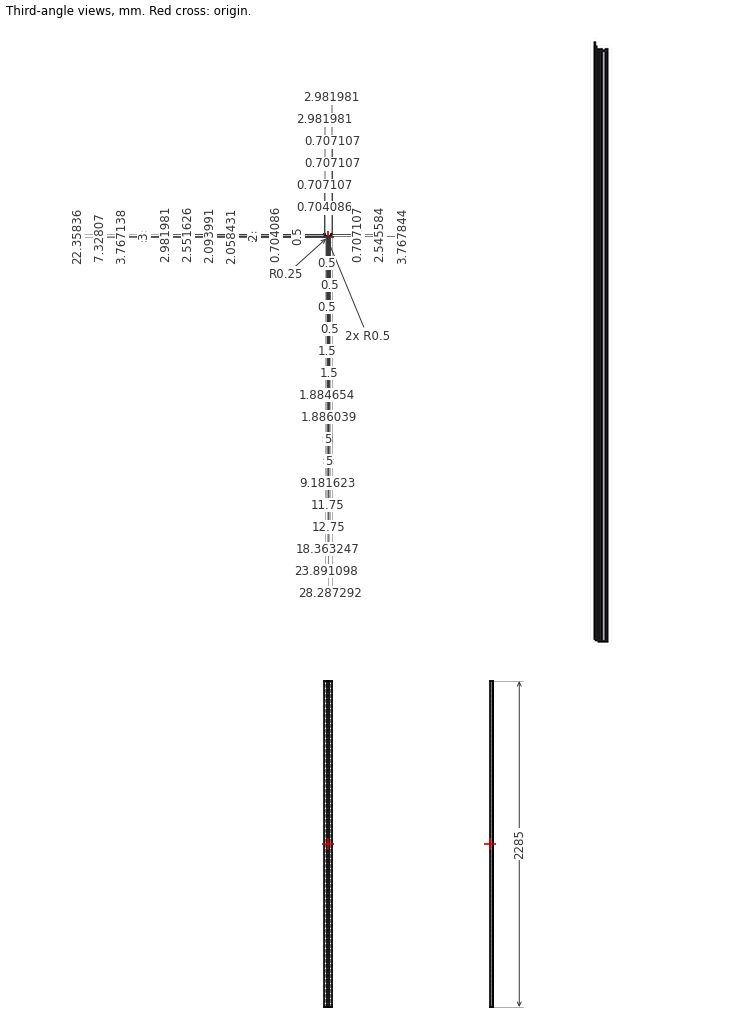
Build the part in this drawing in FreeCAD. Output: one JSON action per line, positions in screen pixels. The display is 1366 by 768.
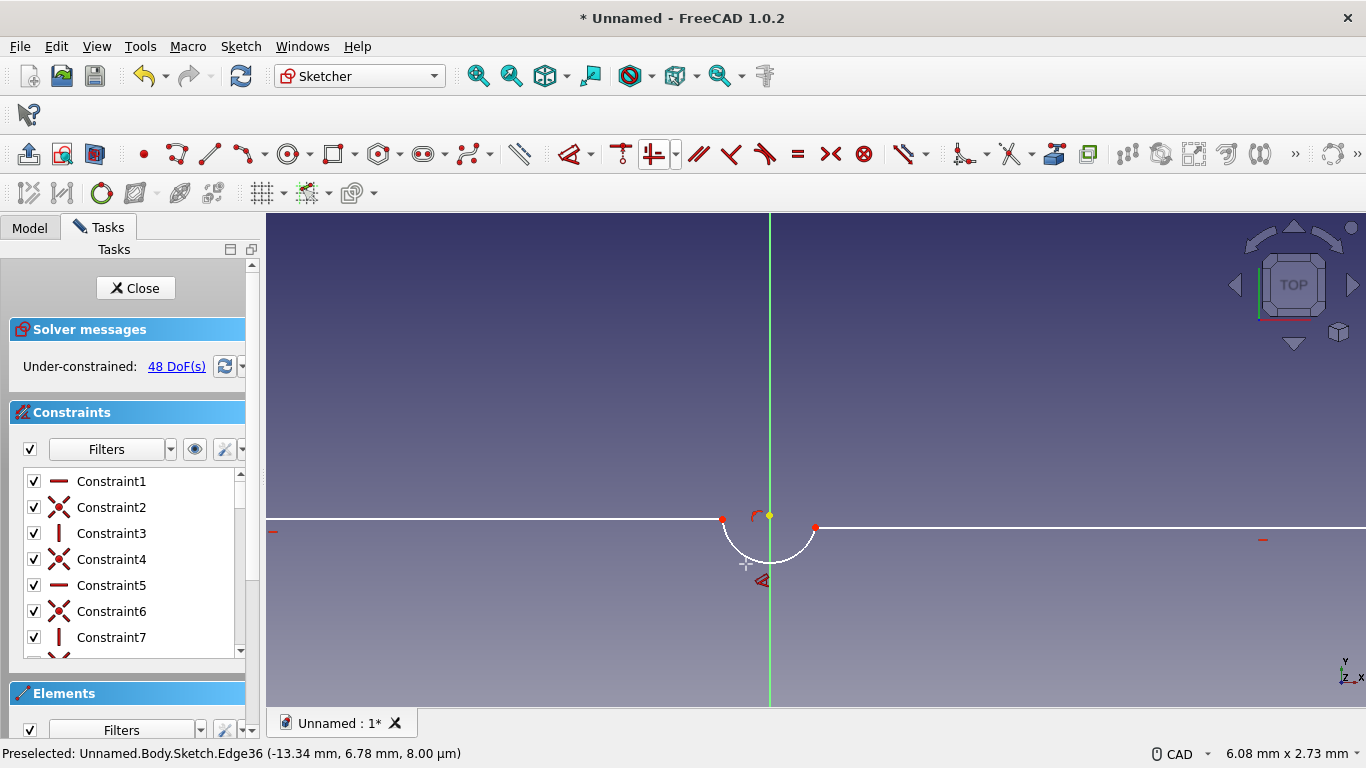
{"action": "left_click", "coordinate": [741, 553]}
{"action": "left_click", "coordinate": [721, 578]}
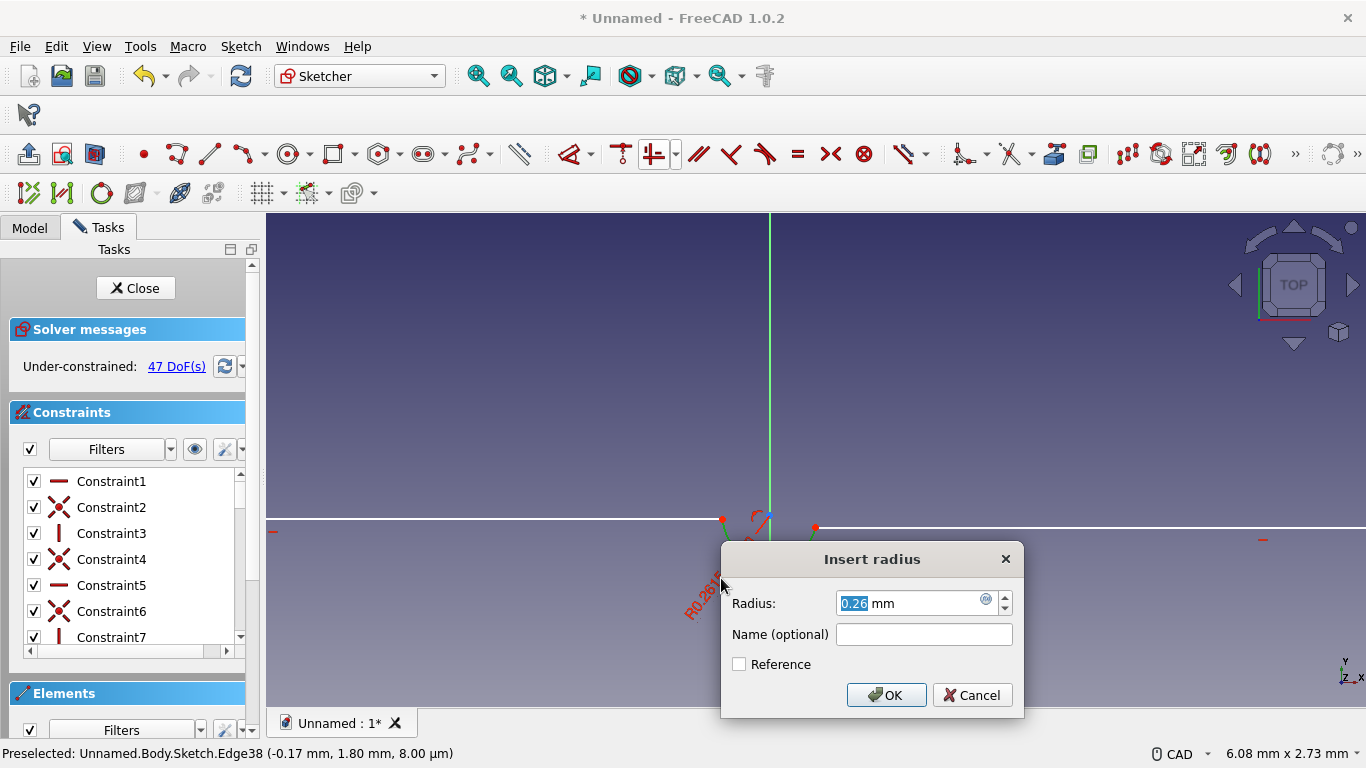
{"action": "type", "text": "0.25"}
{"action": "key", "text": "Return"}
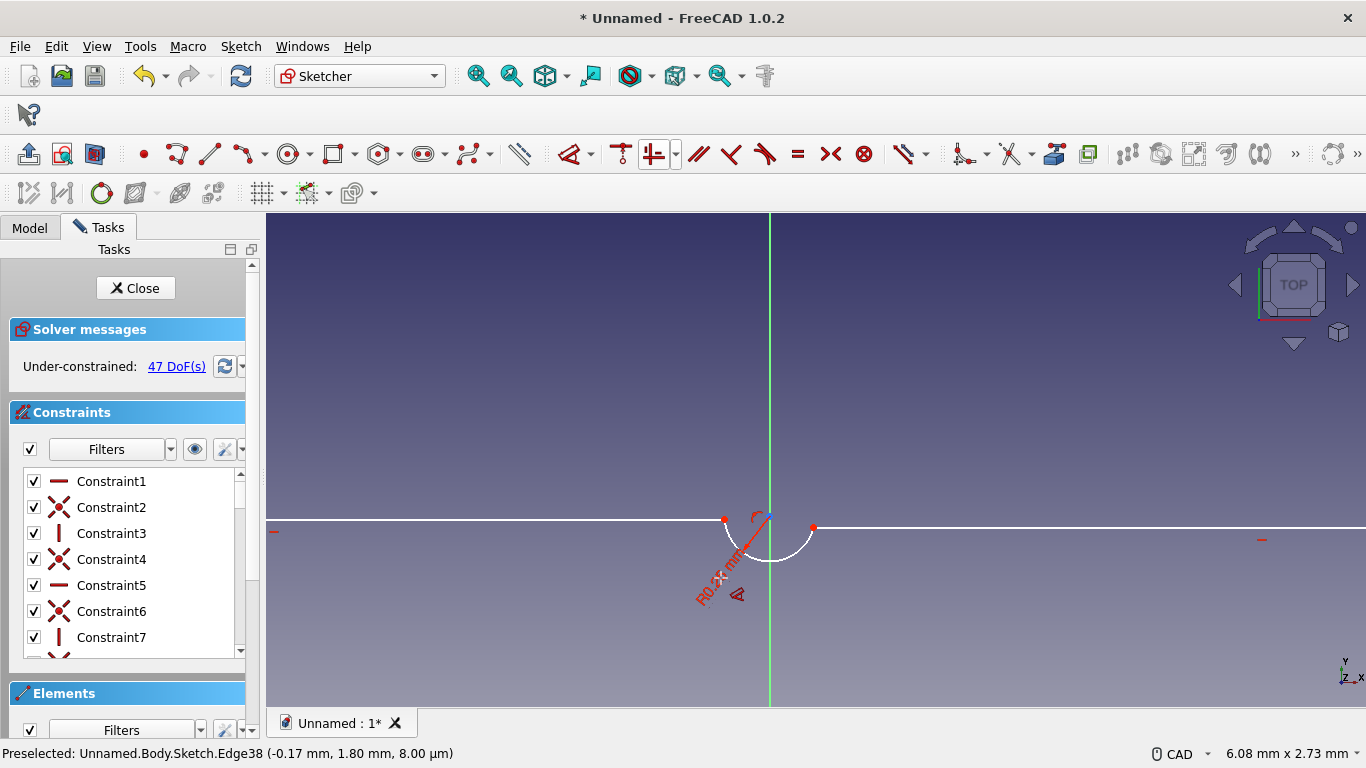
{"action": "scroll", "coordinate": [746, 564], "scroll_direction": "down", "scroll_amount": 14}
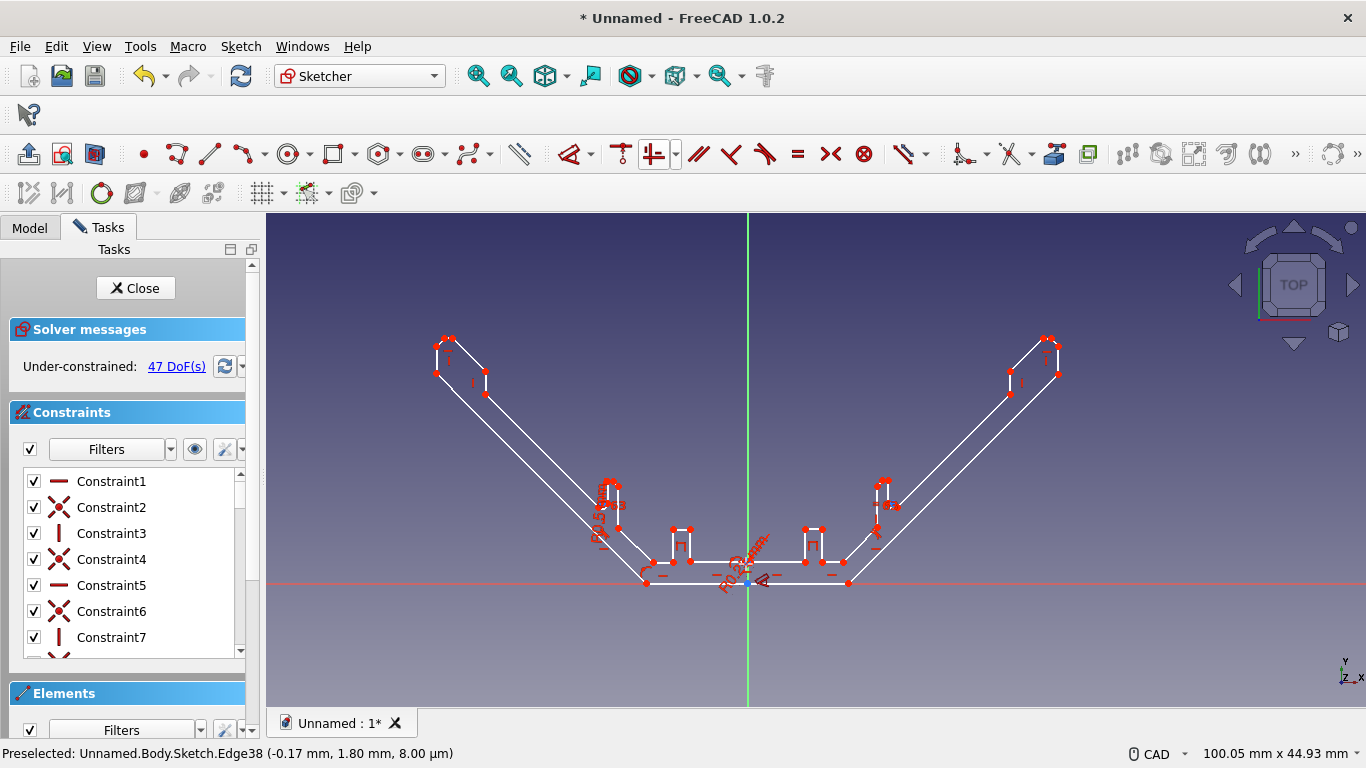
{"action": "left_click", "coordinate": [729, 562]}
{"action": "left_click", "coordinate": [718, 528]}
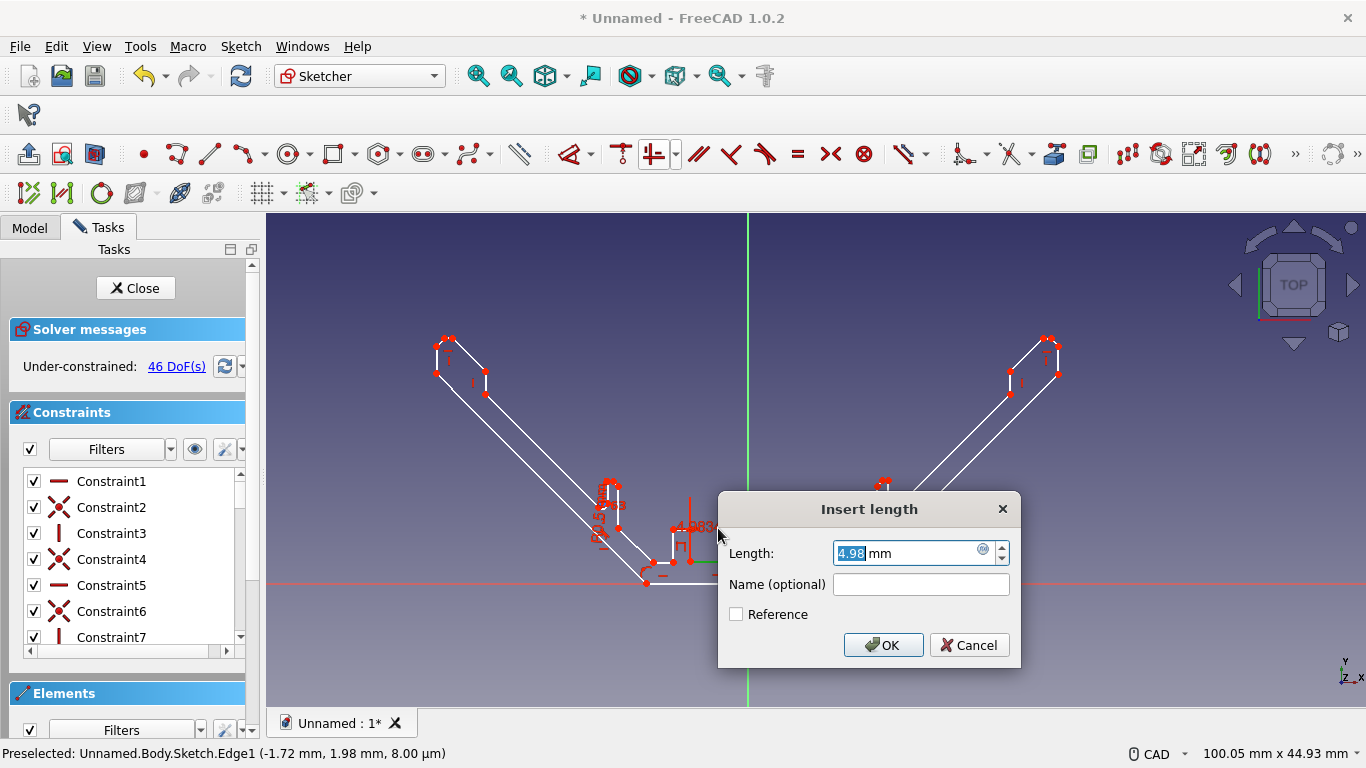
{"action": "type", "text": "5"}
{"action": "key", "text": "Return"}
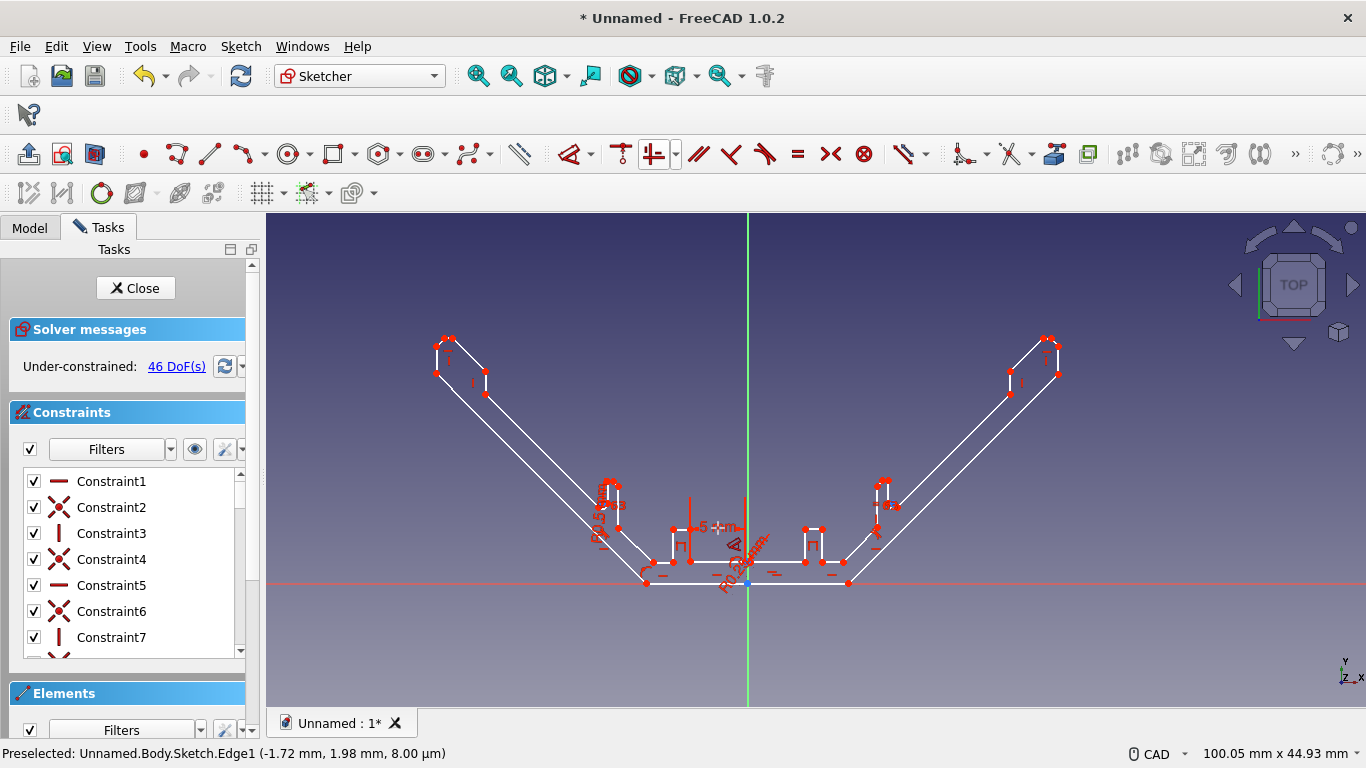
{"action": "scroll", "coordinate": [690, 552], "scroll_direction": "up", "scroll_amount": 2}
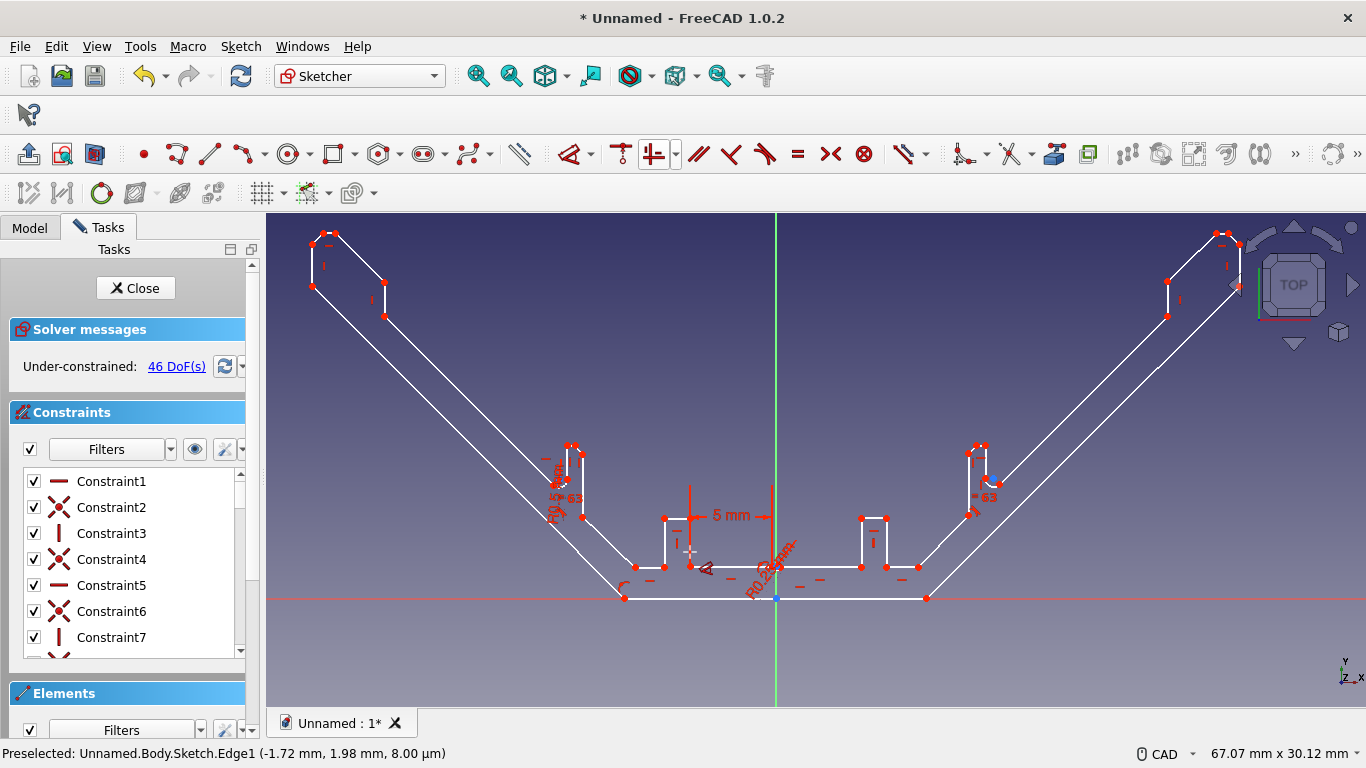
{"action": "left_click", "coordinate": [690, 552]}
{"action": "left_click", "coordinate": [724, 543]}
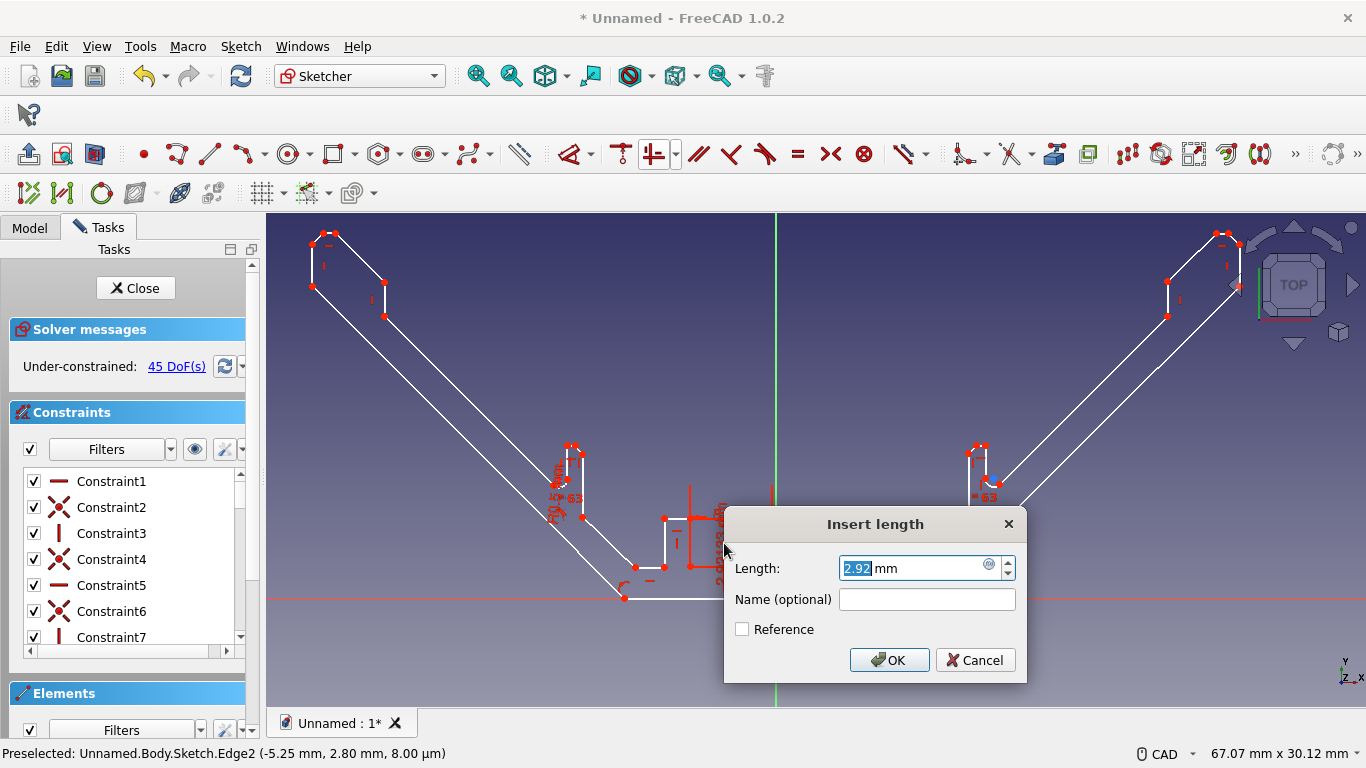
{"action": "type", "text": "3"}
{"action": "key", "text": "Return"}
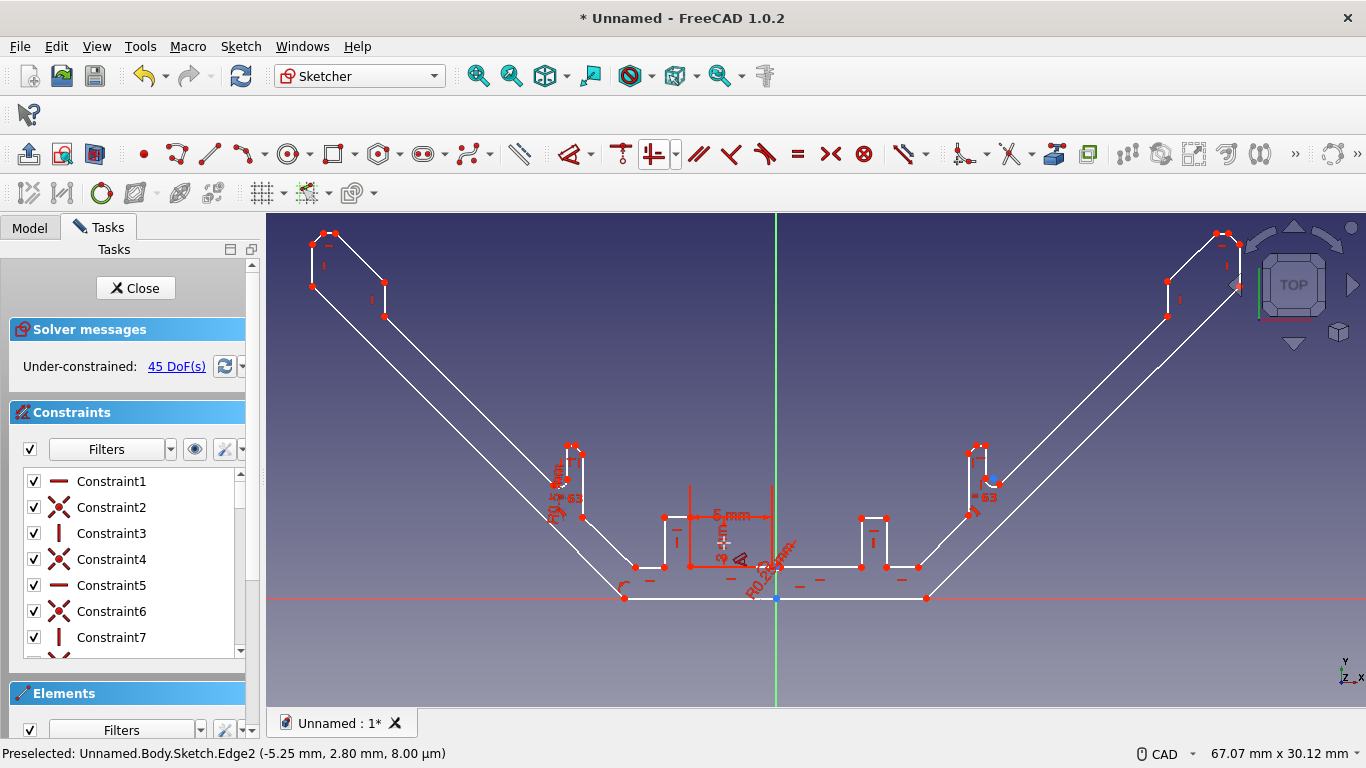
{"action": "left_click", "coordinate": [665, 532]}
{"action": "left_click", "coordinate": [631, 543]}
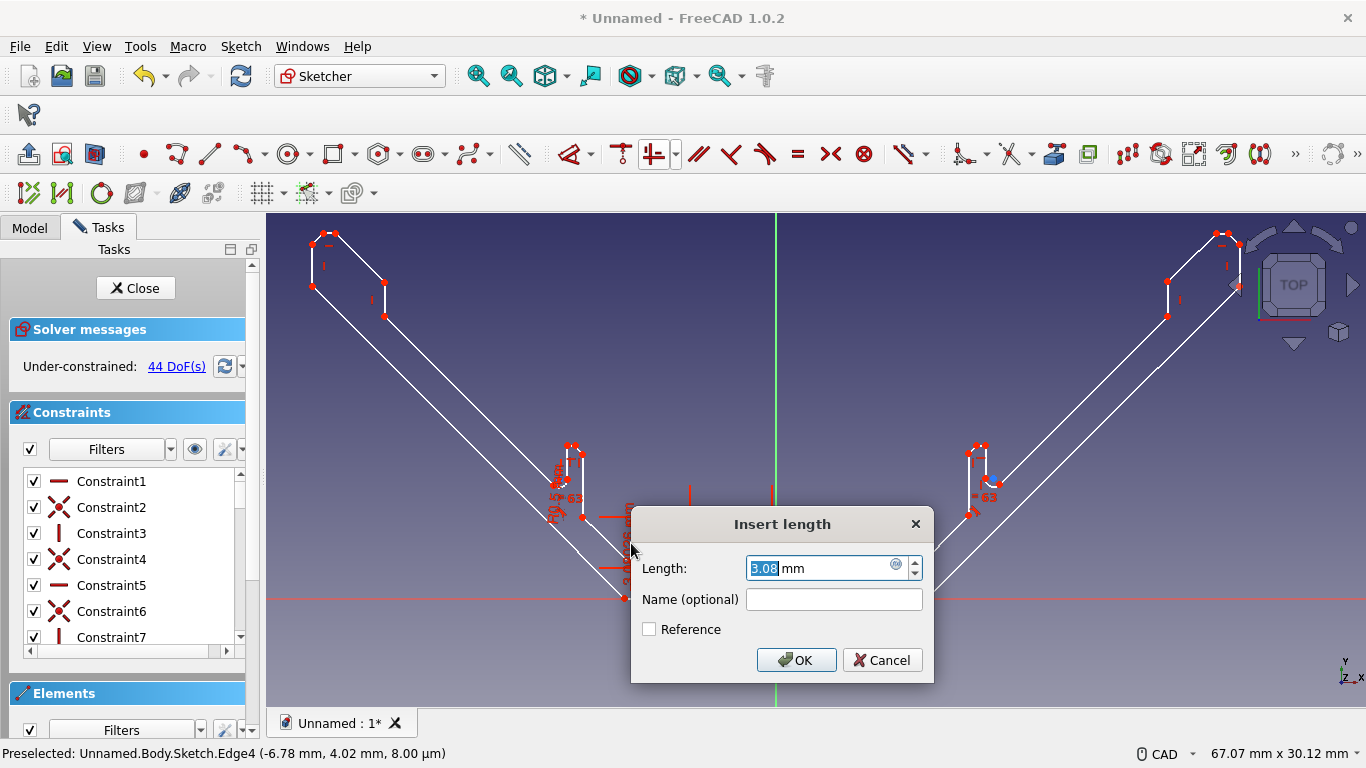
{"action": "type", "text": "3"}
{"action": "key", "text": "Return"}